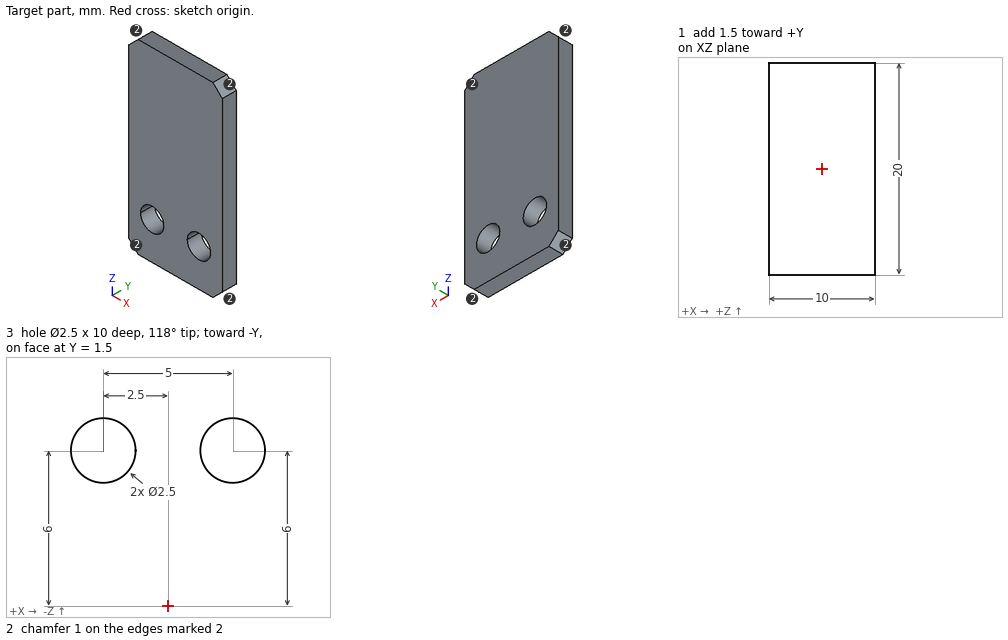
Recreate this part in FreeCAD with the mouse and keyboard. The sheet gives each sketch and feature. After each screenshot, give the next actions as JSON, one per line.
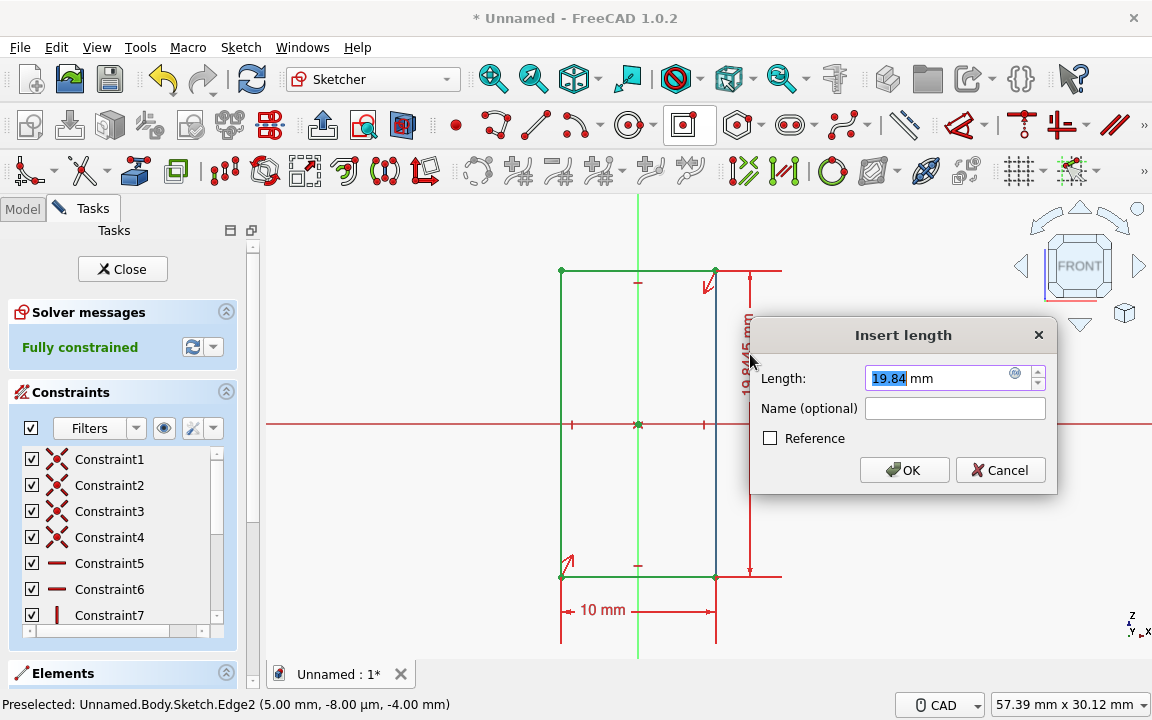
{"action": "type", "text": "20"}
{"action": "key", "text": "Return"}
{"action": "key", "text": "Escape"}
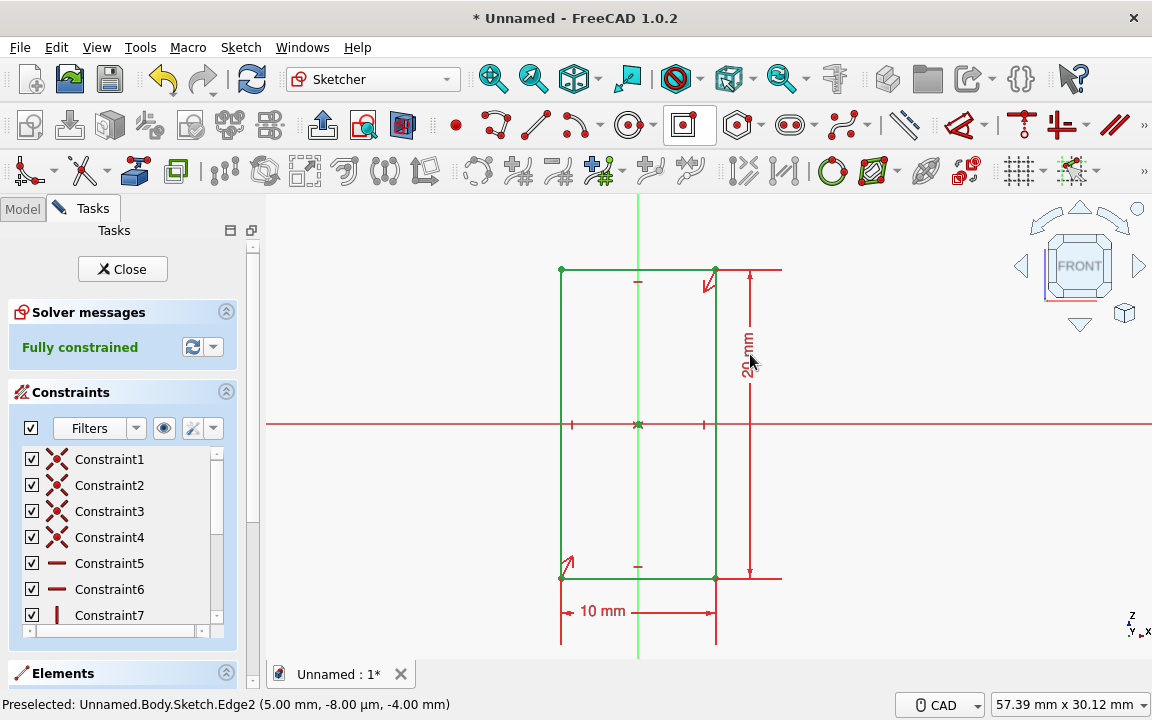
{"action": "left_click", "coordinate": [123, 269]}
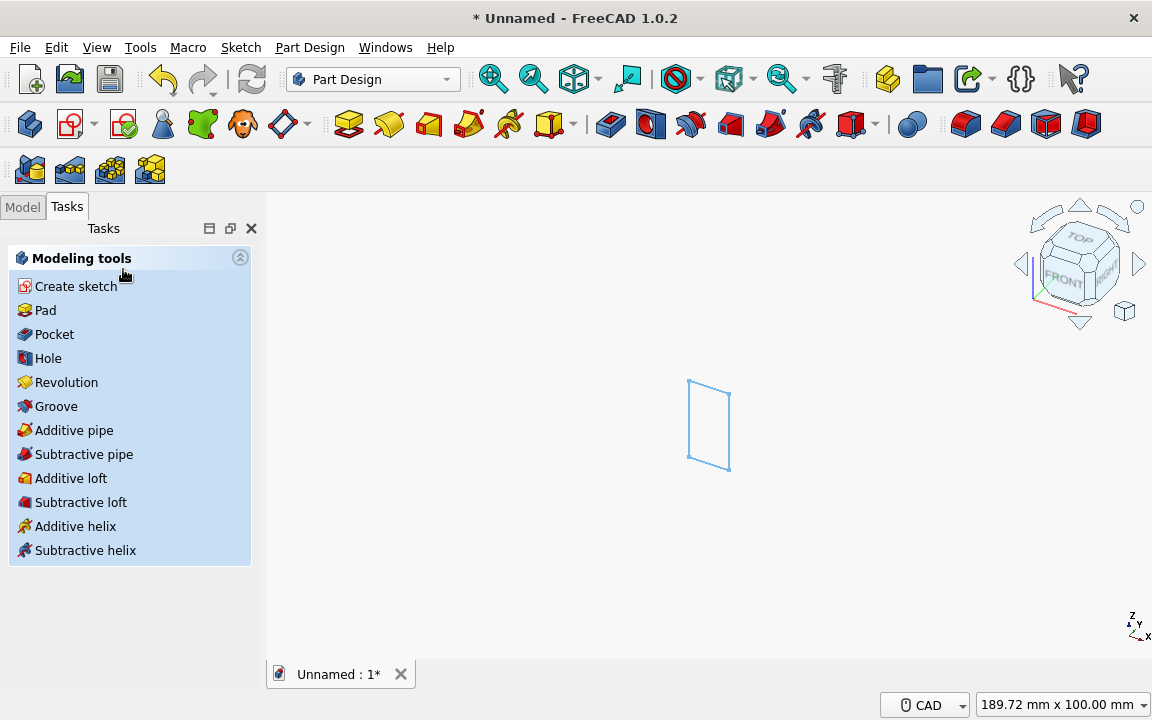
{"action": "left_click", "coordinate": [350, 124]}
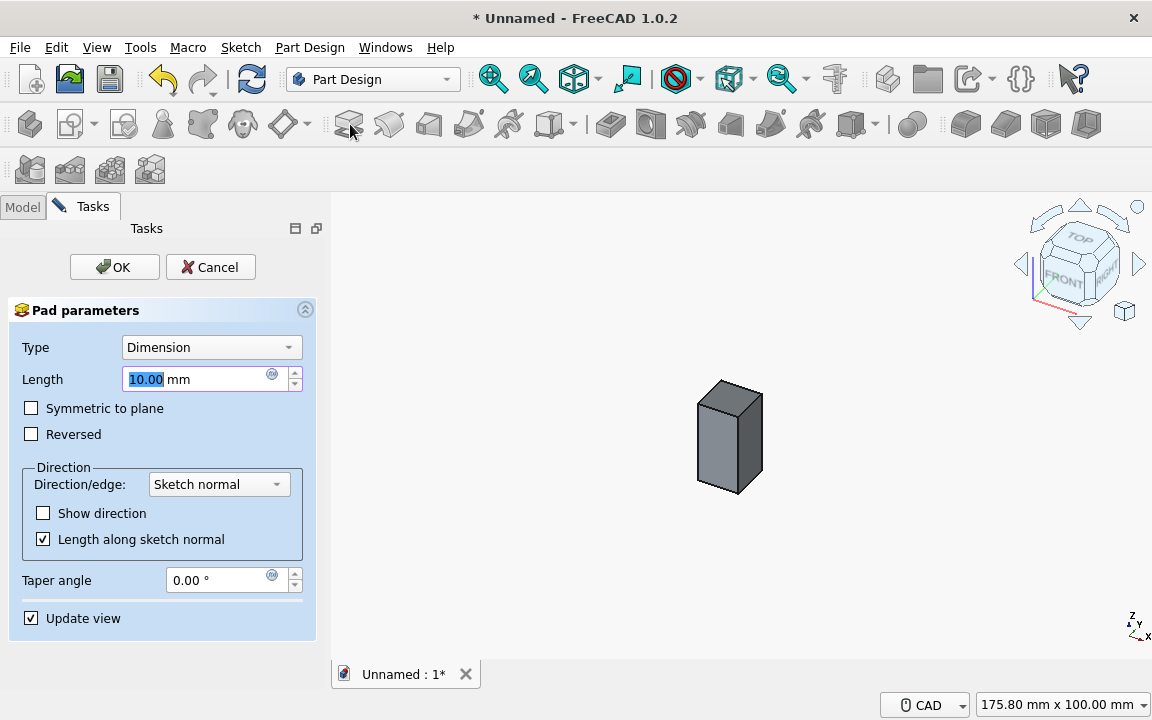
{"action": "type", "text": "1.5"}
{"action": "key", "text": "Tab"}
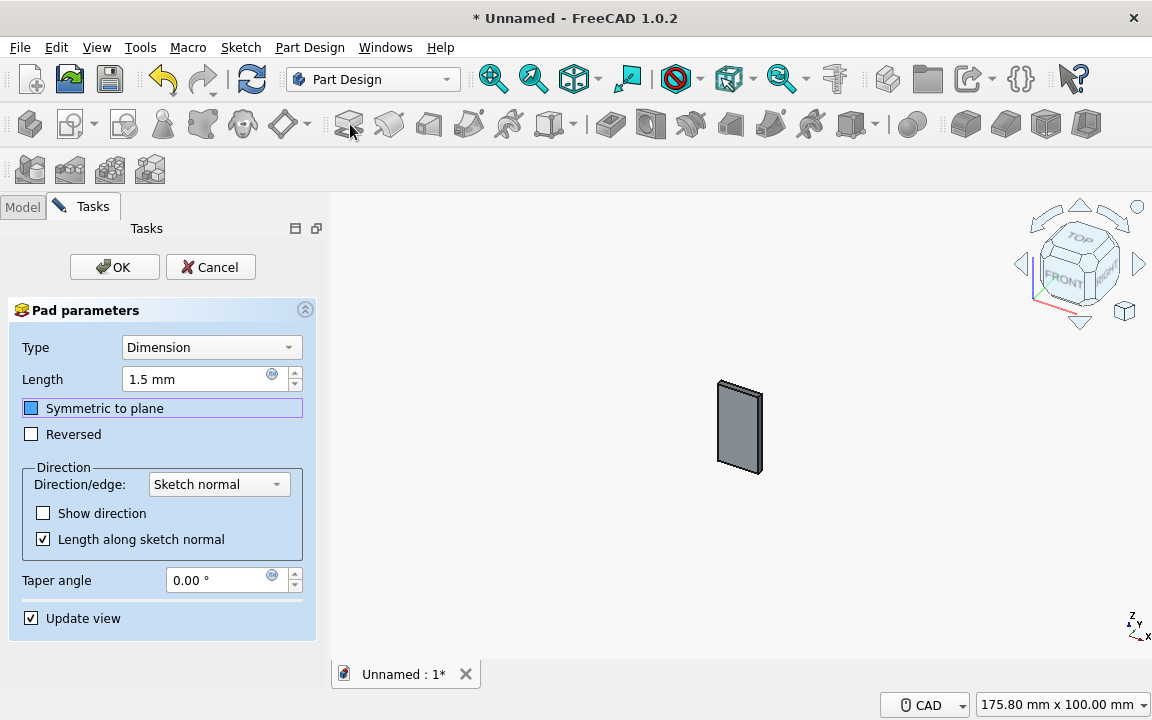
{"action": "left_click", "coordinate": [30, 434]}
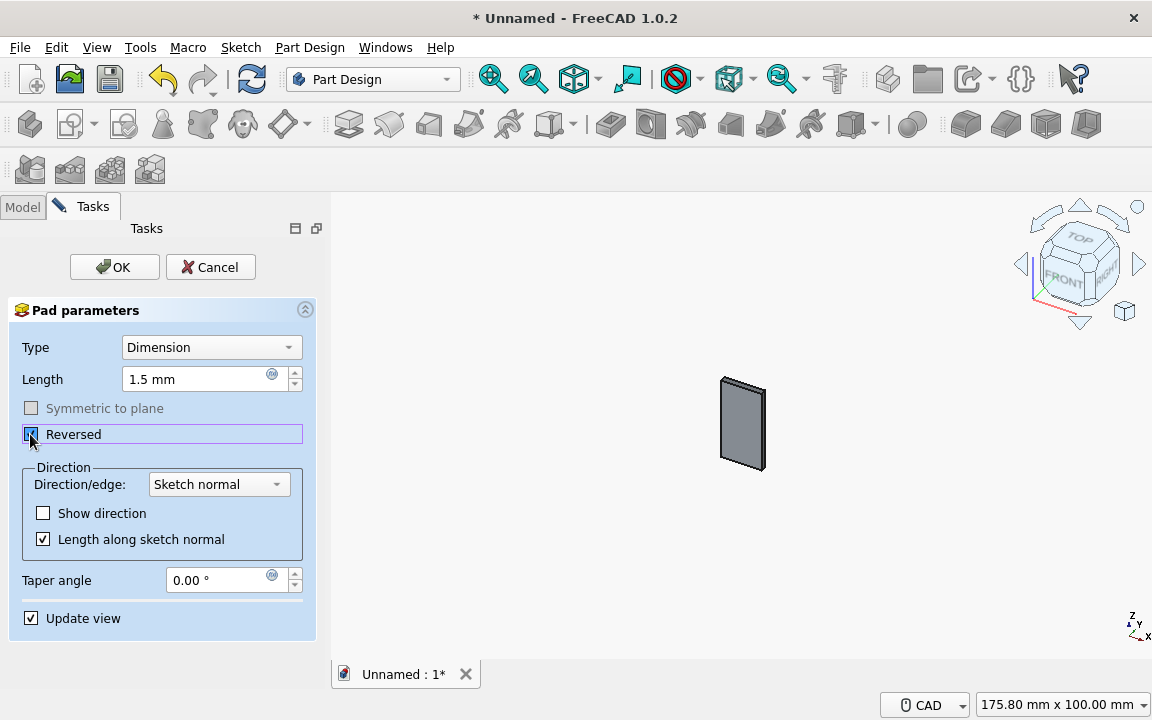
{"action": "left_click", "coordinate": [115, 267]}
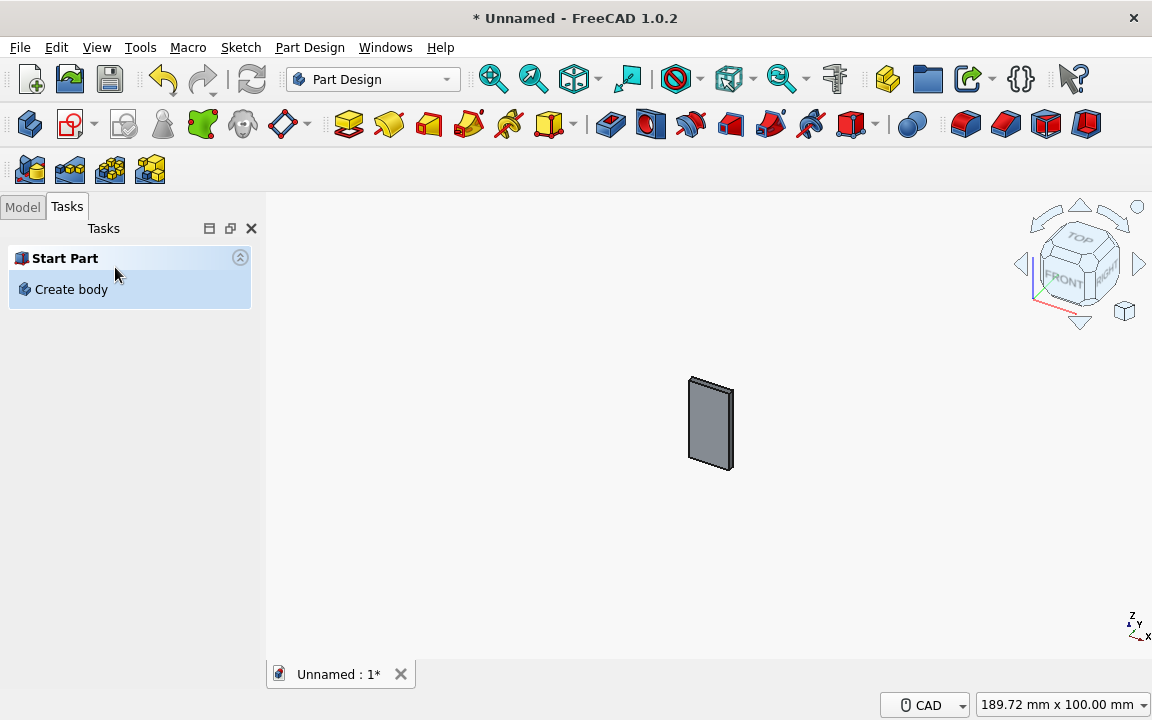
{"action": "key", "text": "v f"}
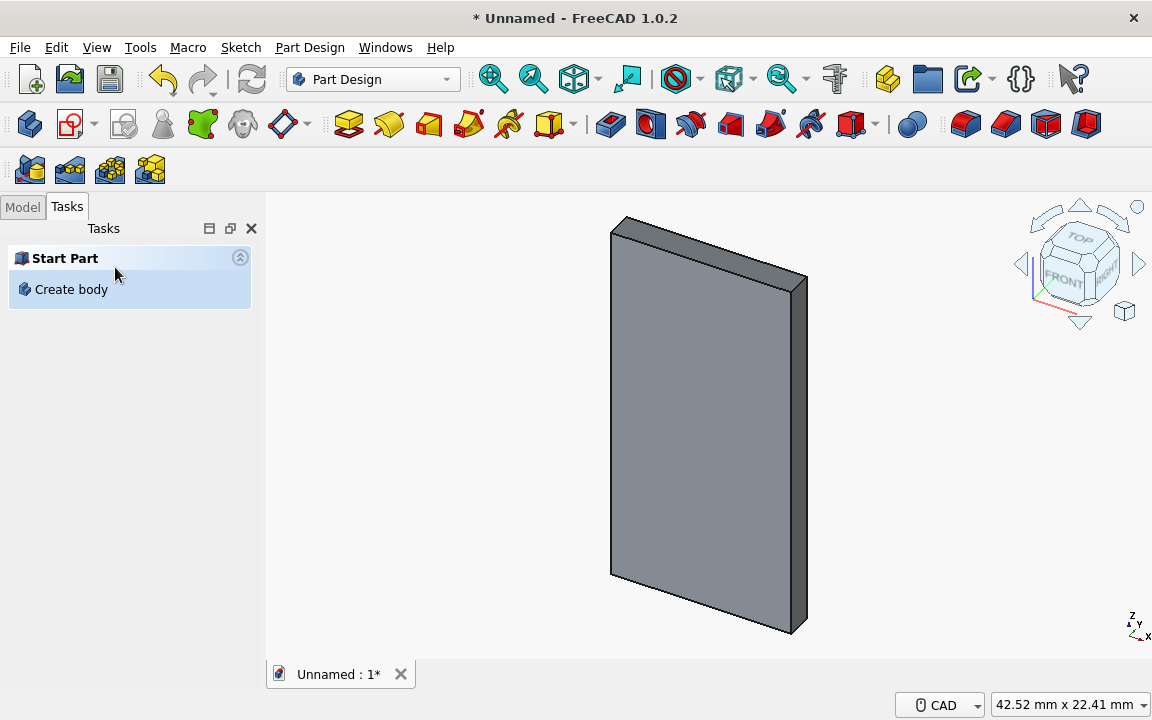
{"action": "left_click", "coordinate": [799, 284]}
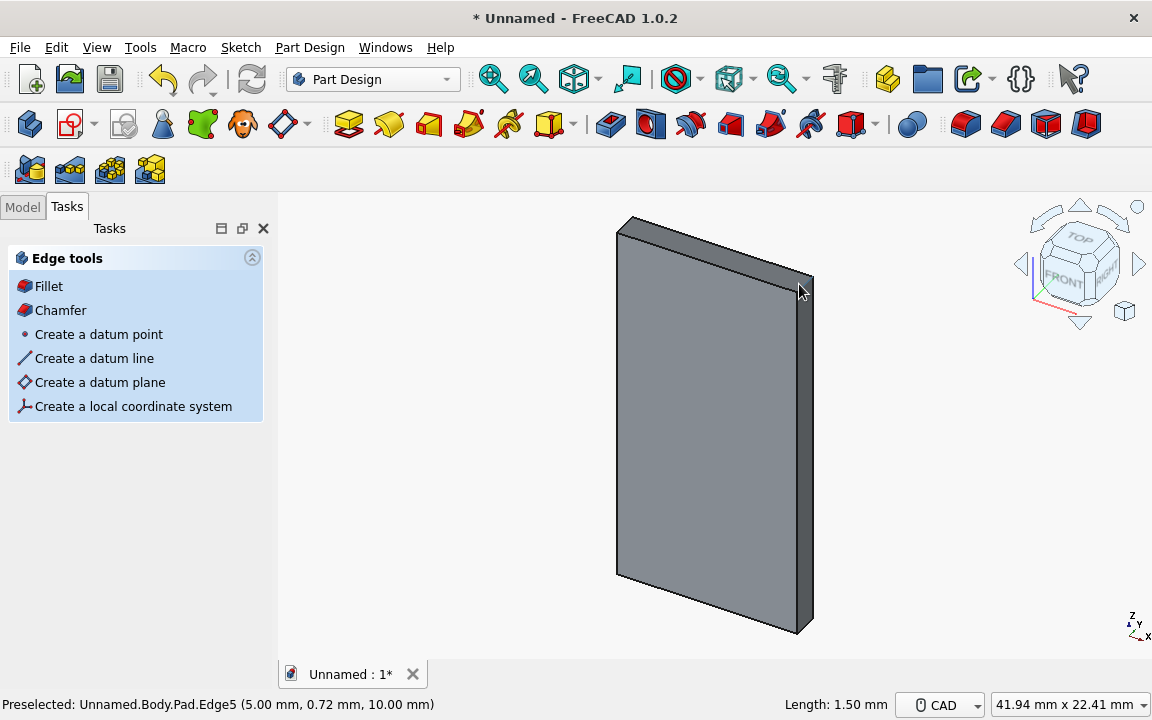
{"action": "key", "text": "0"}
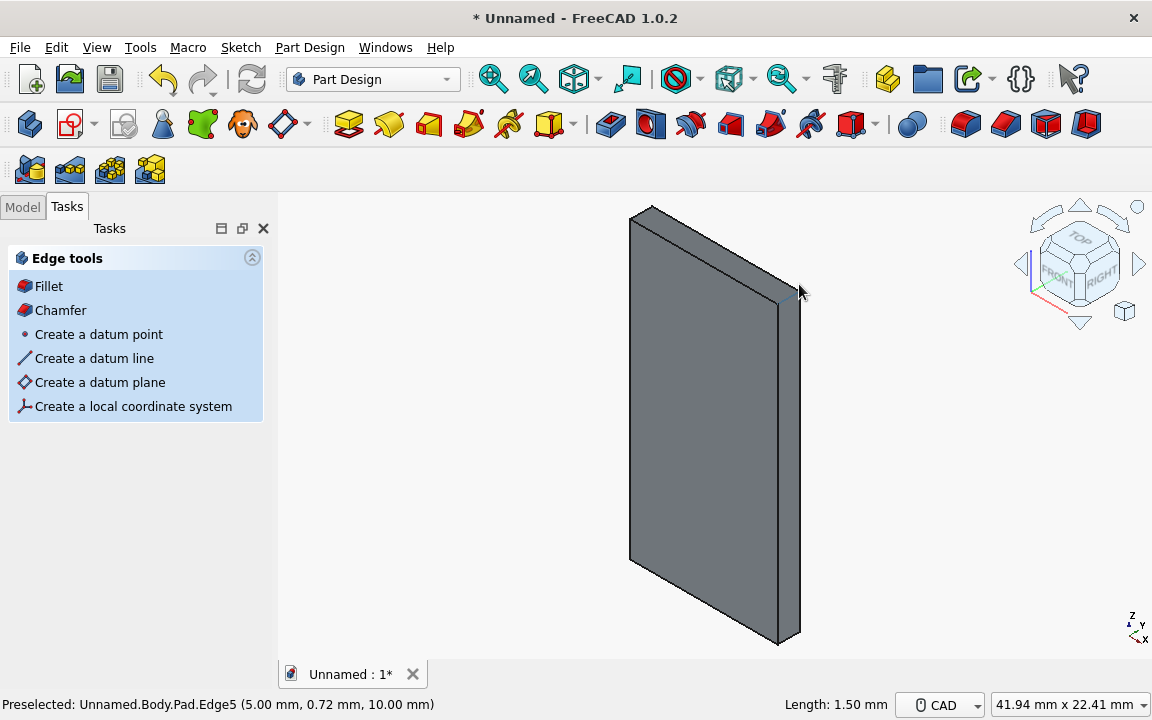
{"action": "key", "text": "2"}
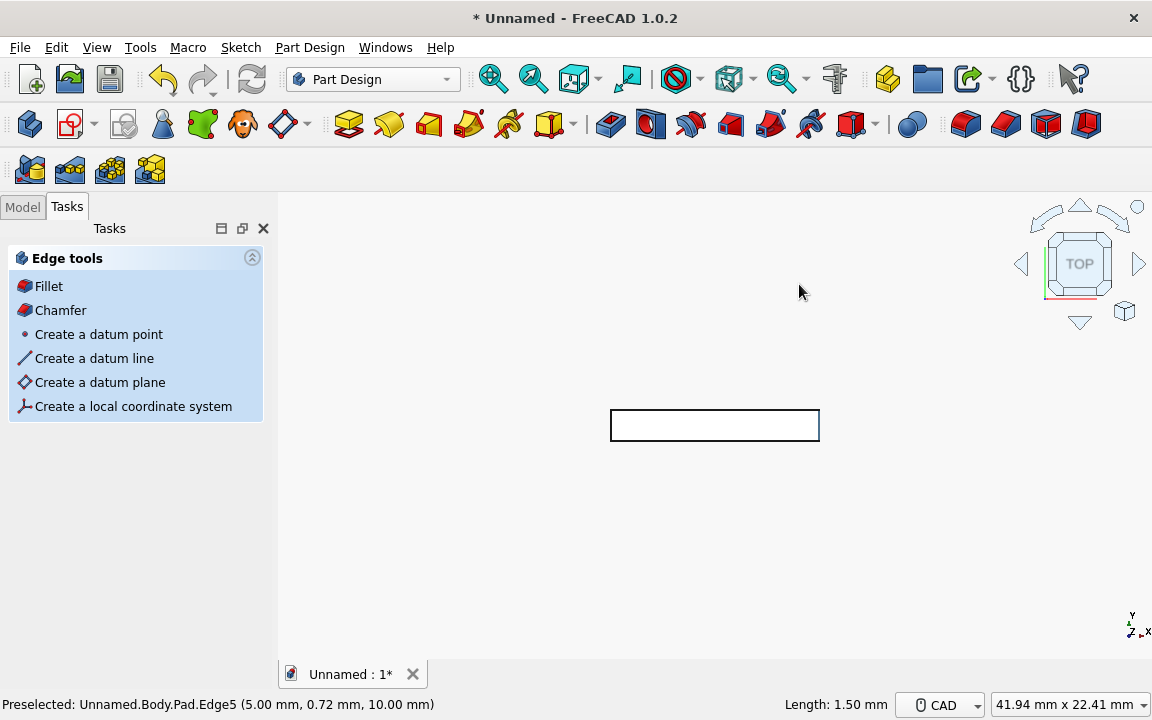
{"action": "left_click", "coordinate": [494, 80]}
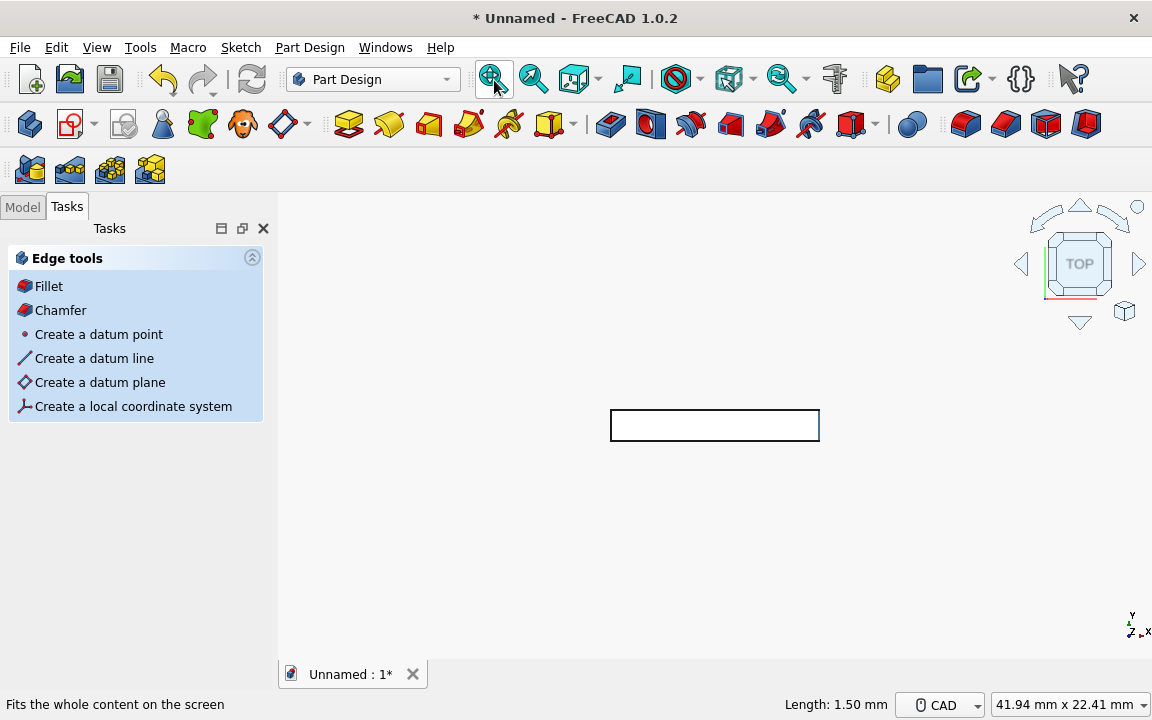
{"action": "left_click", "coordinate": [611, 424], "text": "ctrl"}